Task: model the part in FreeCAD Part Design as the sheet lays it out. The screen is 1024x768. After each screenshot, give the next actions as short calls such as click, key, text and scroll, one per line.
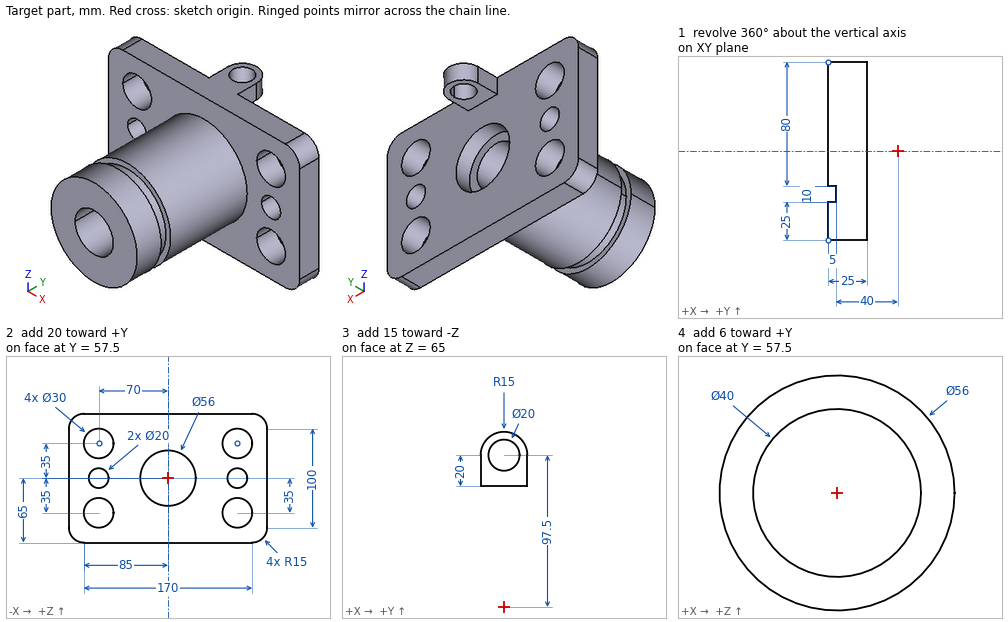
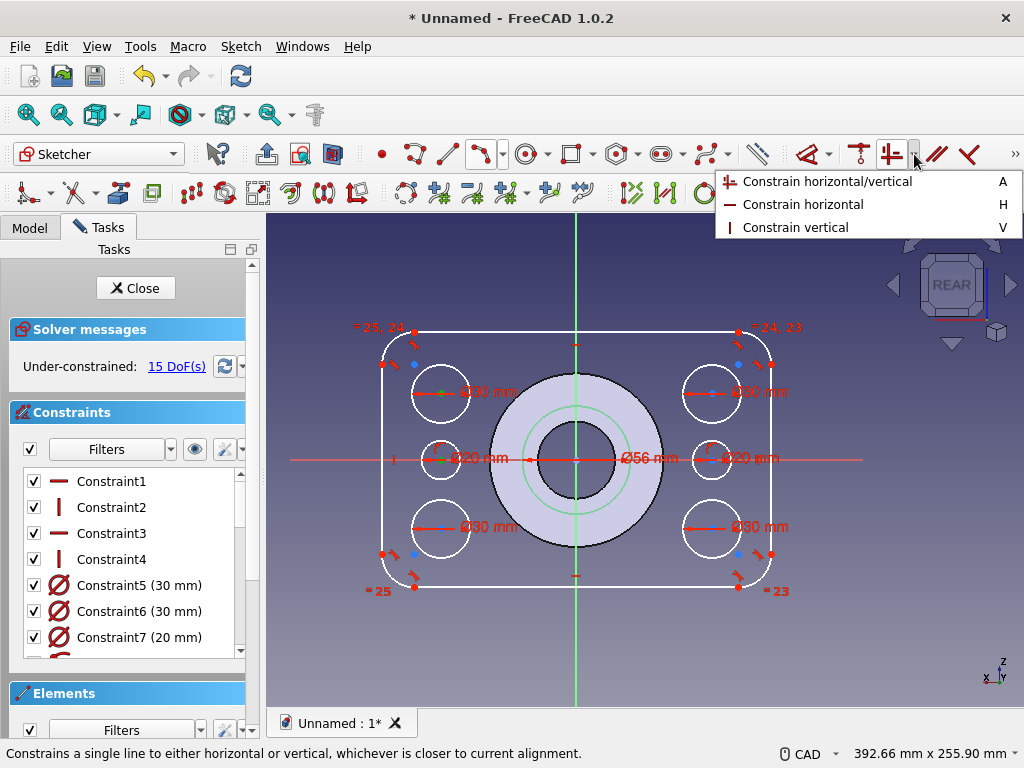
click(869, 228)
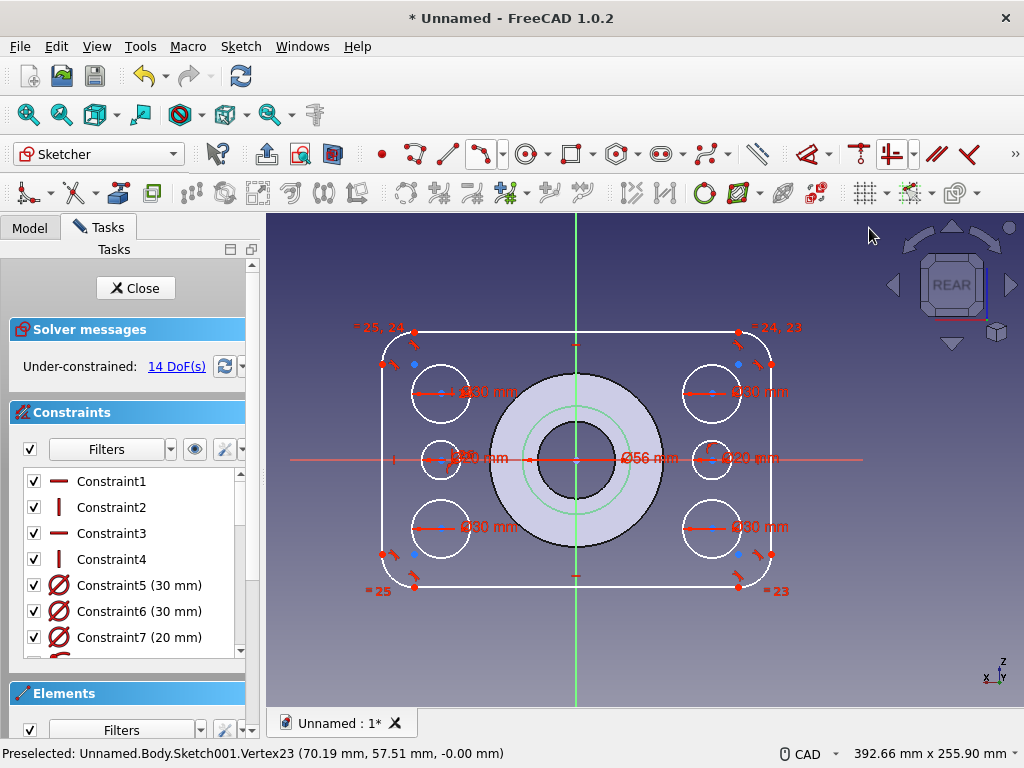
click(441, 460)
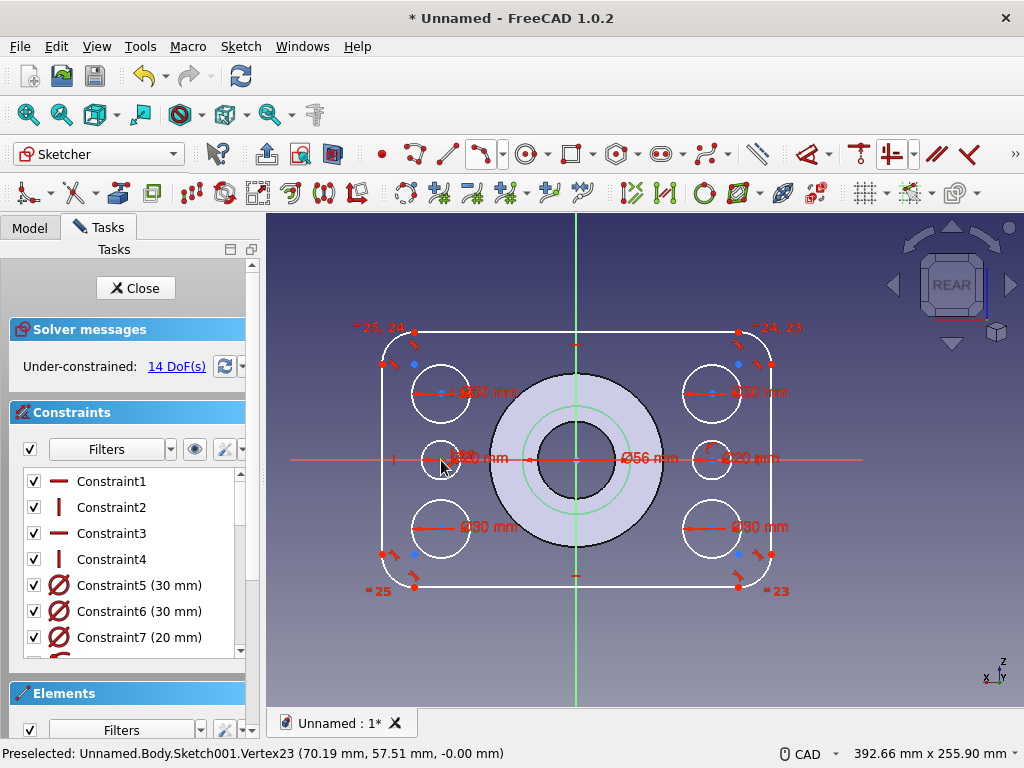
click(441, 529)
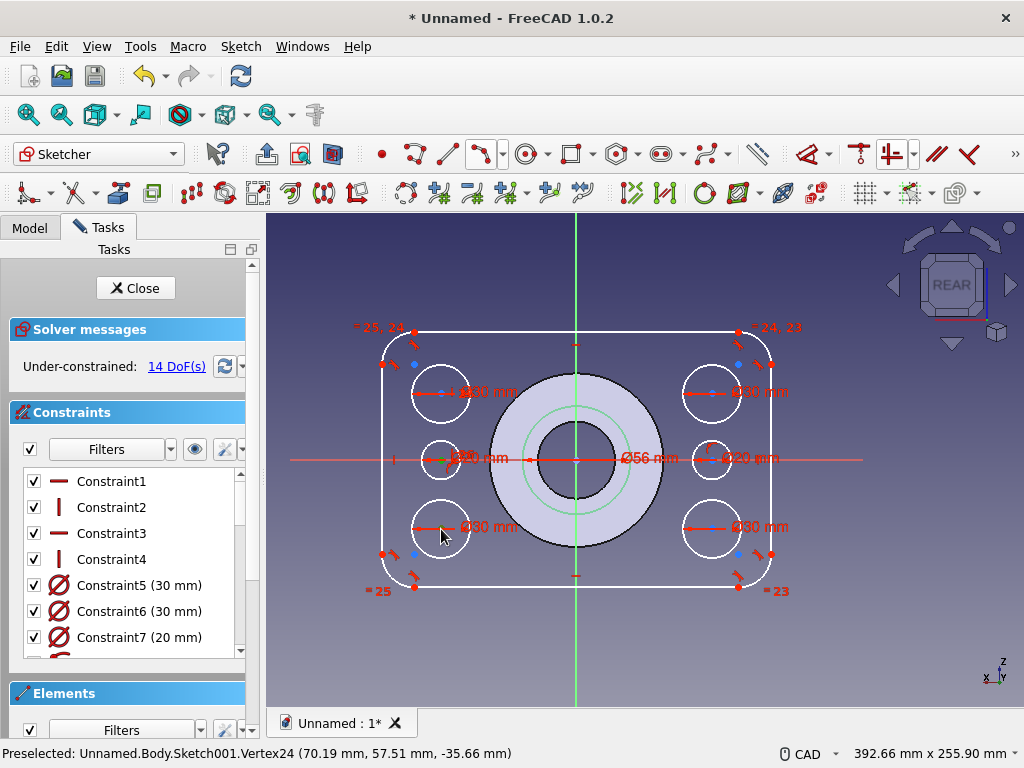
click(914, 154)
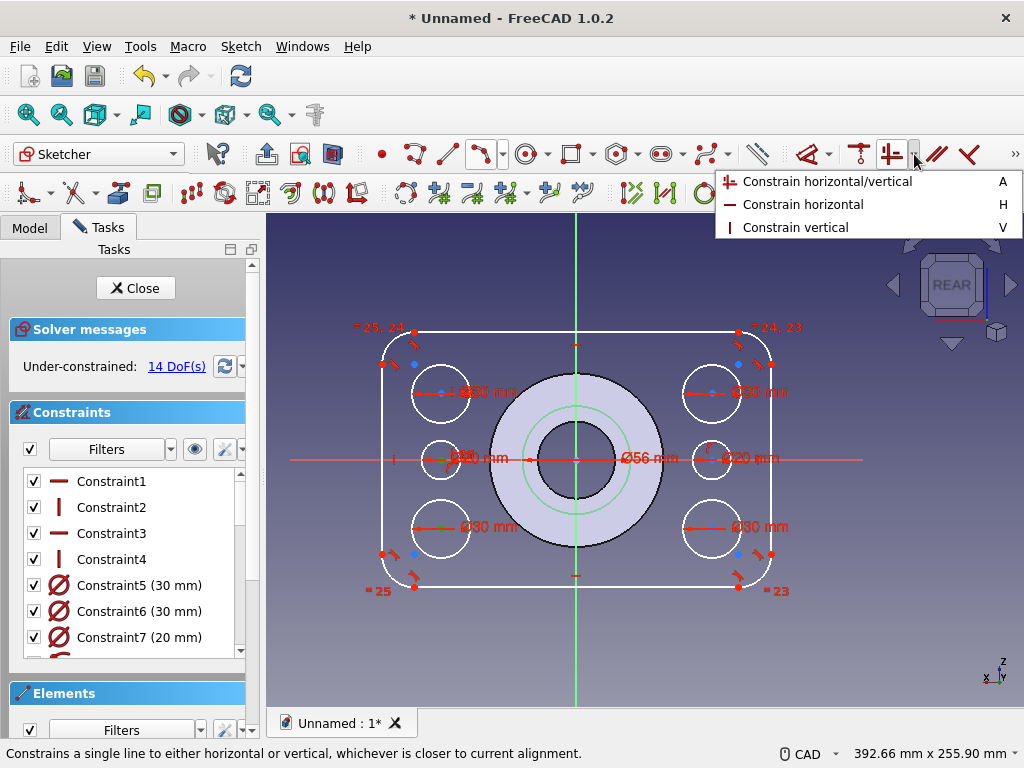
click(869, 228)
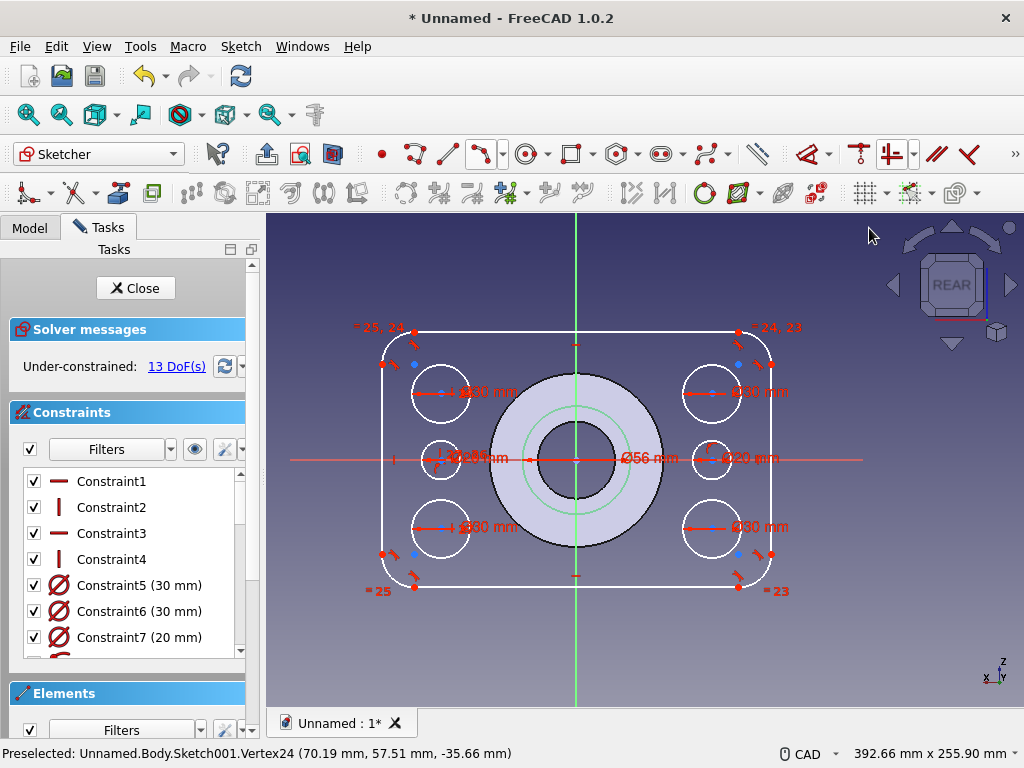
click(712, 394)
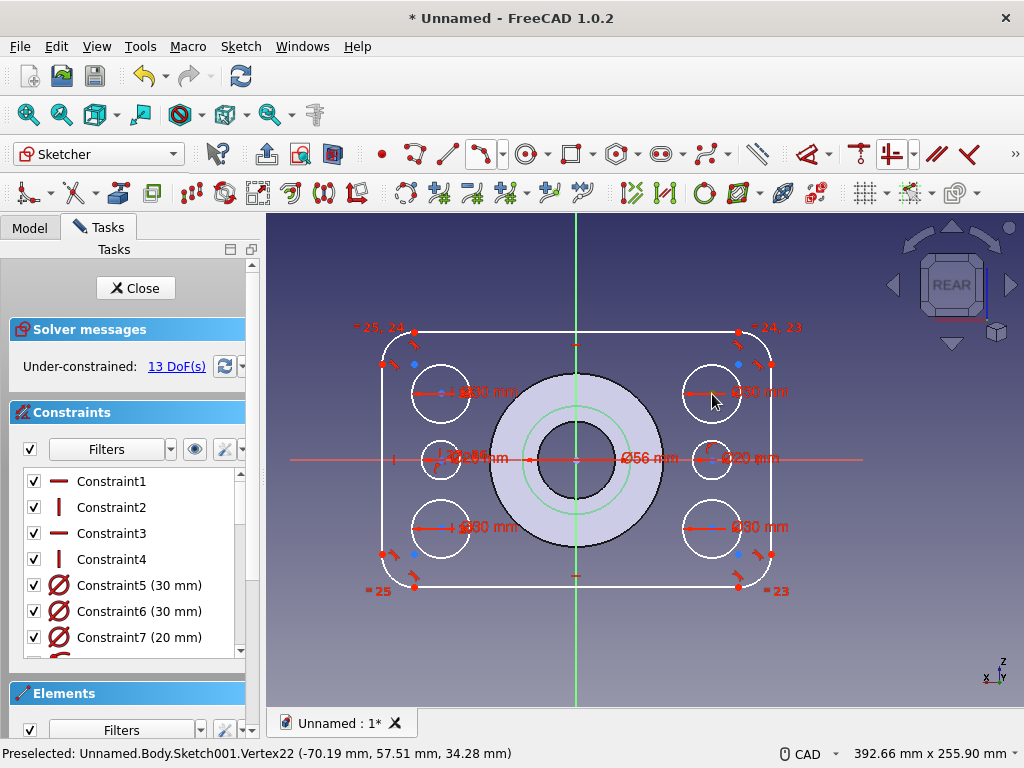
click(712, 460)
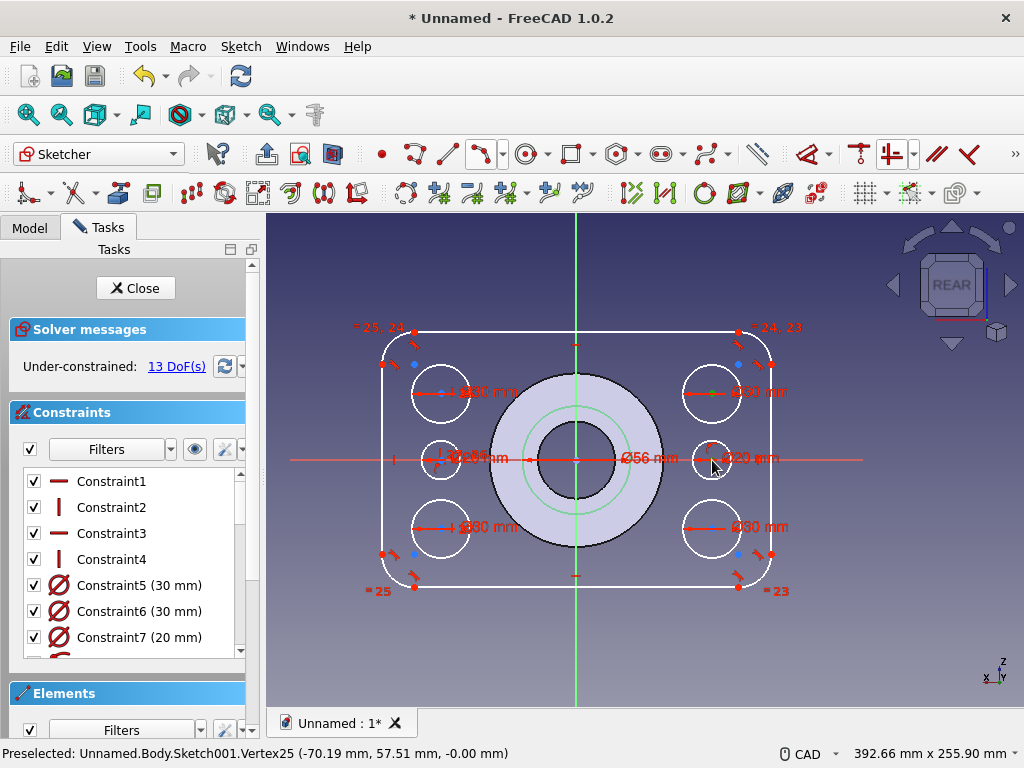
key(v)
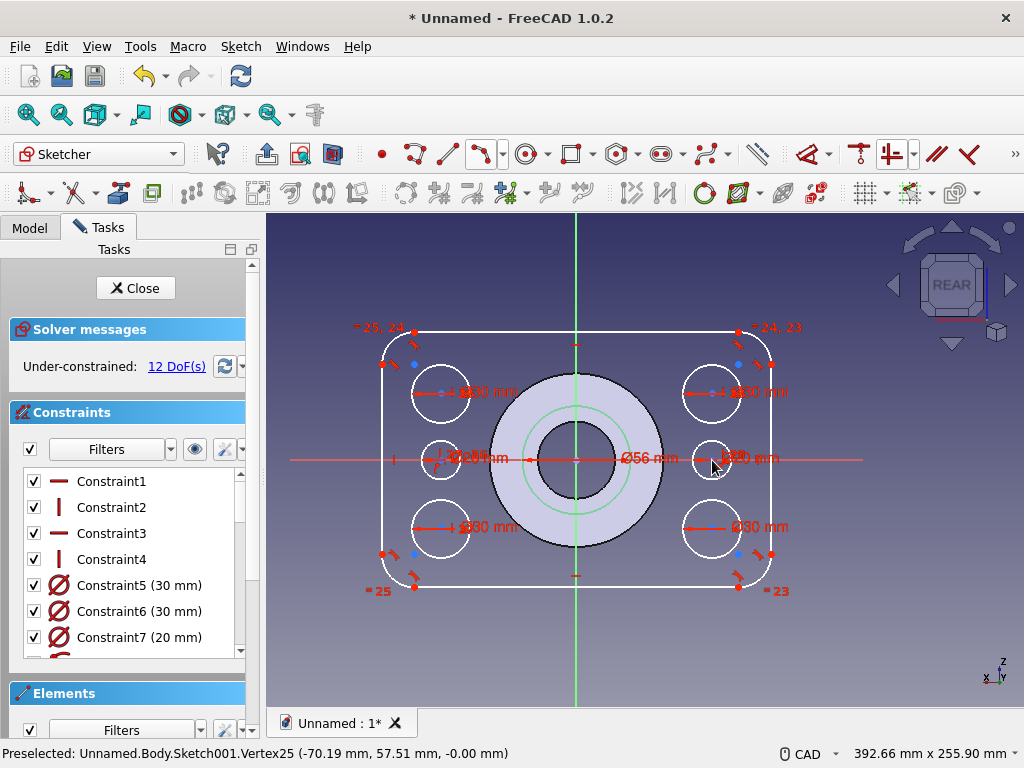
click(712, 460)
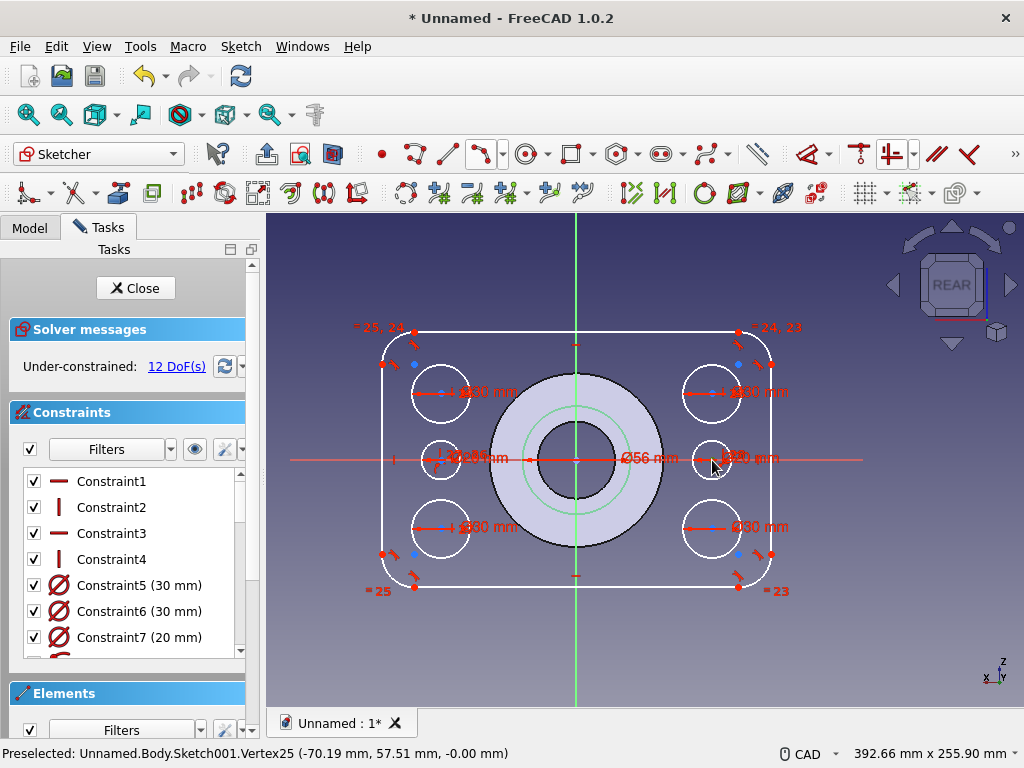
click(712, 529)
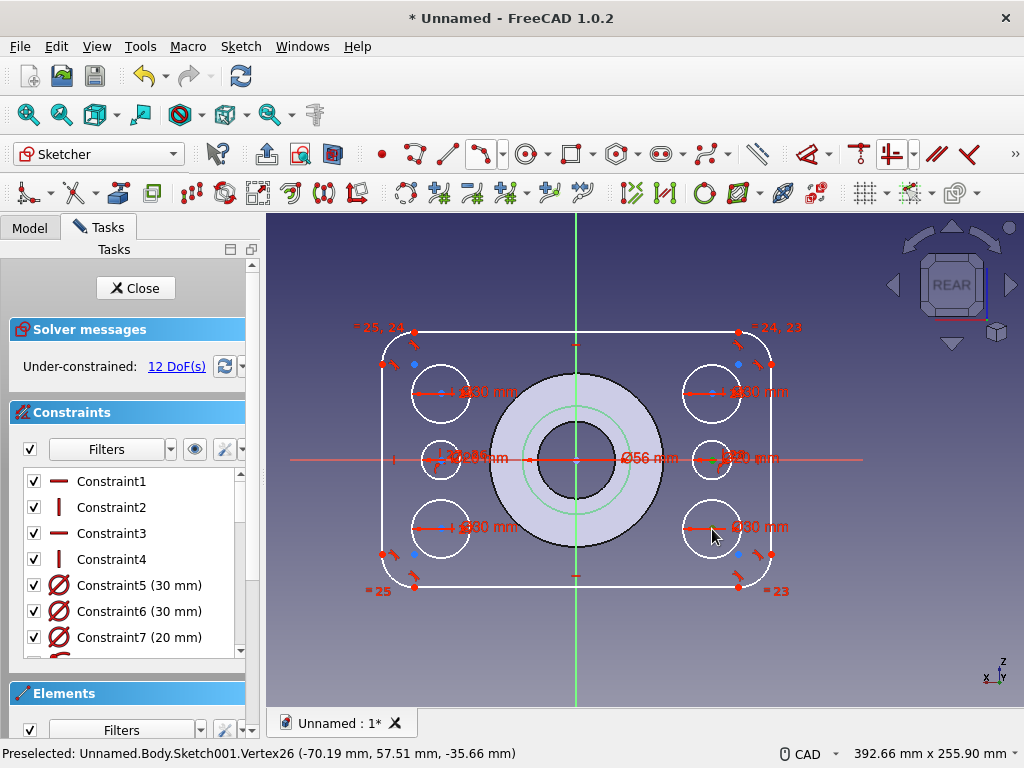
click(914, 154)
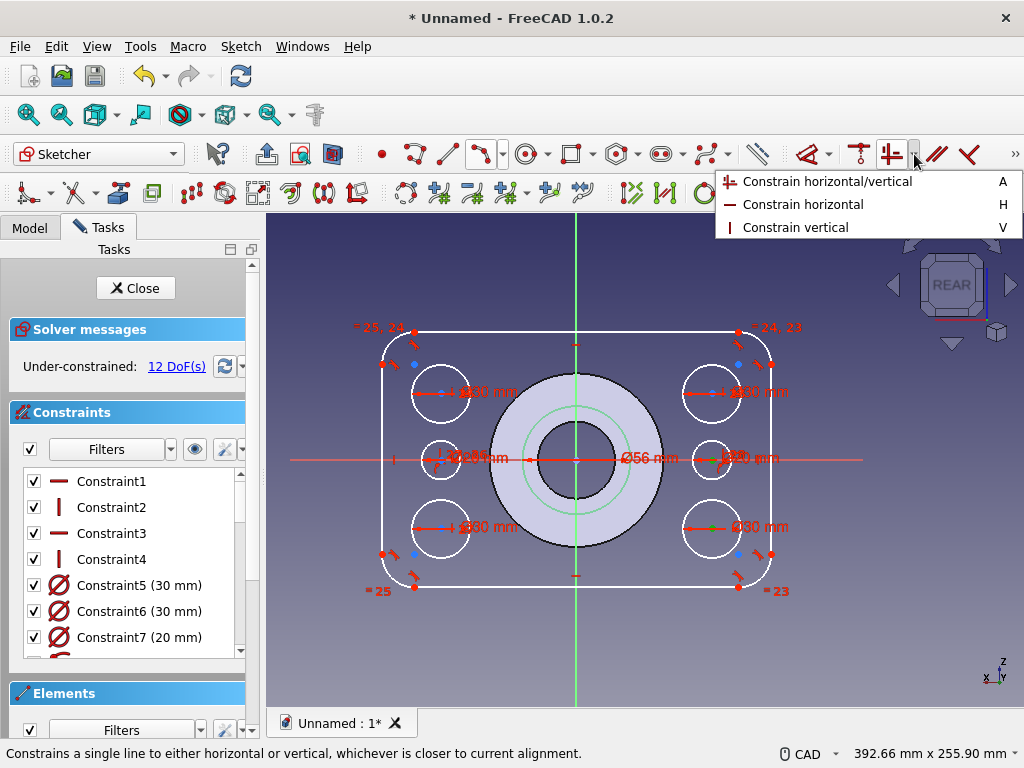
click(869, 228)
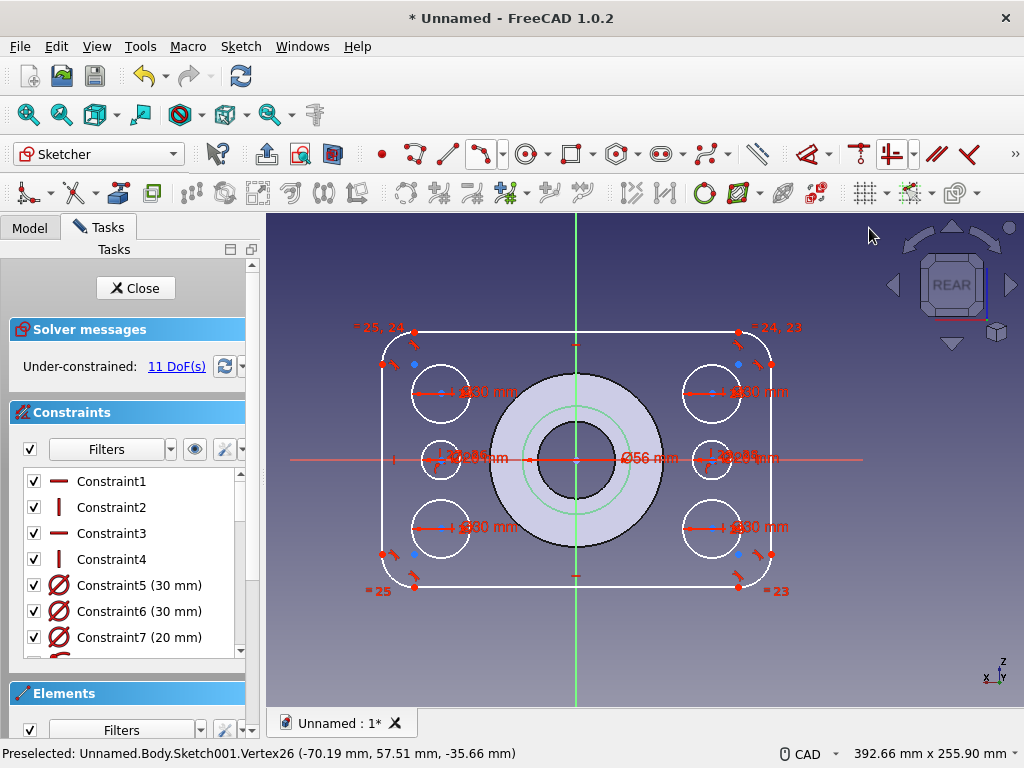
click(441, 394)